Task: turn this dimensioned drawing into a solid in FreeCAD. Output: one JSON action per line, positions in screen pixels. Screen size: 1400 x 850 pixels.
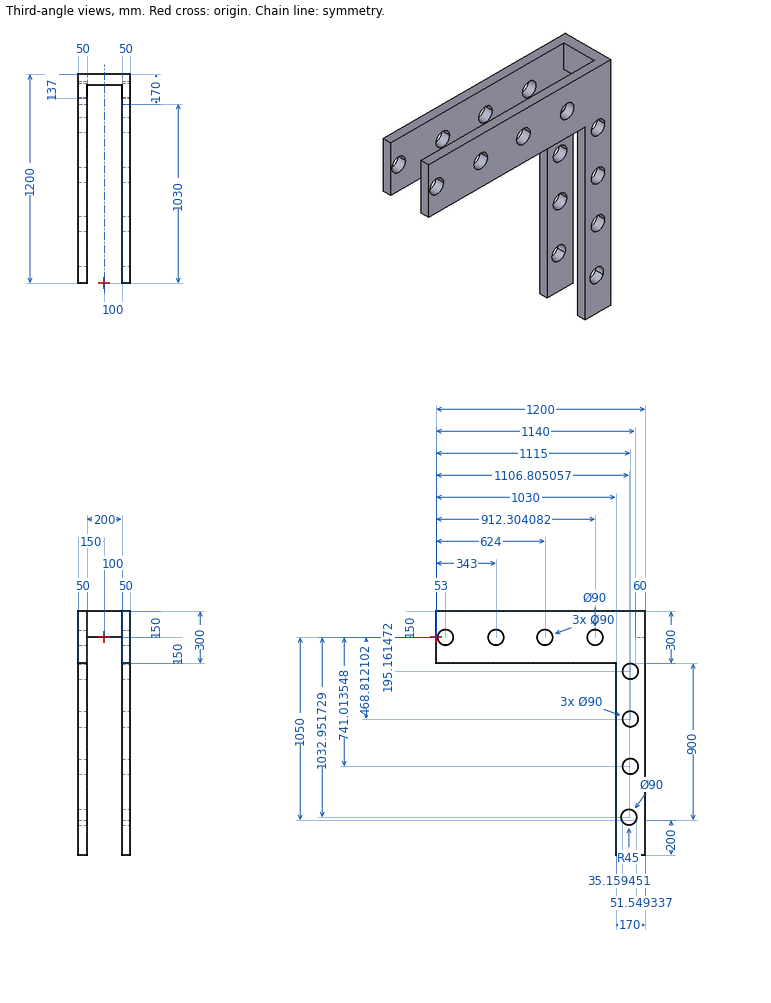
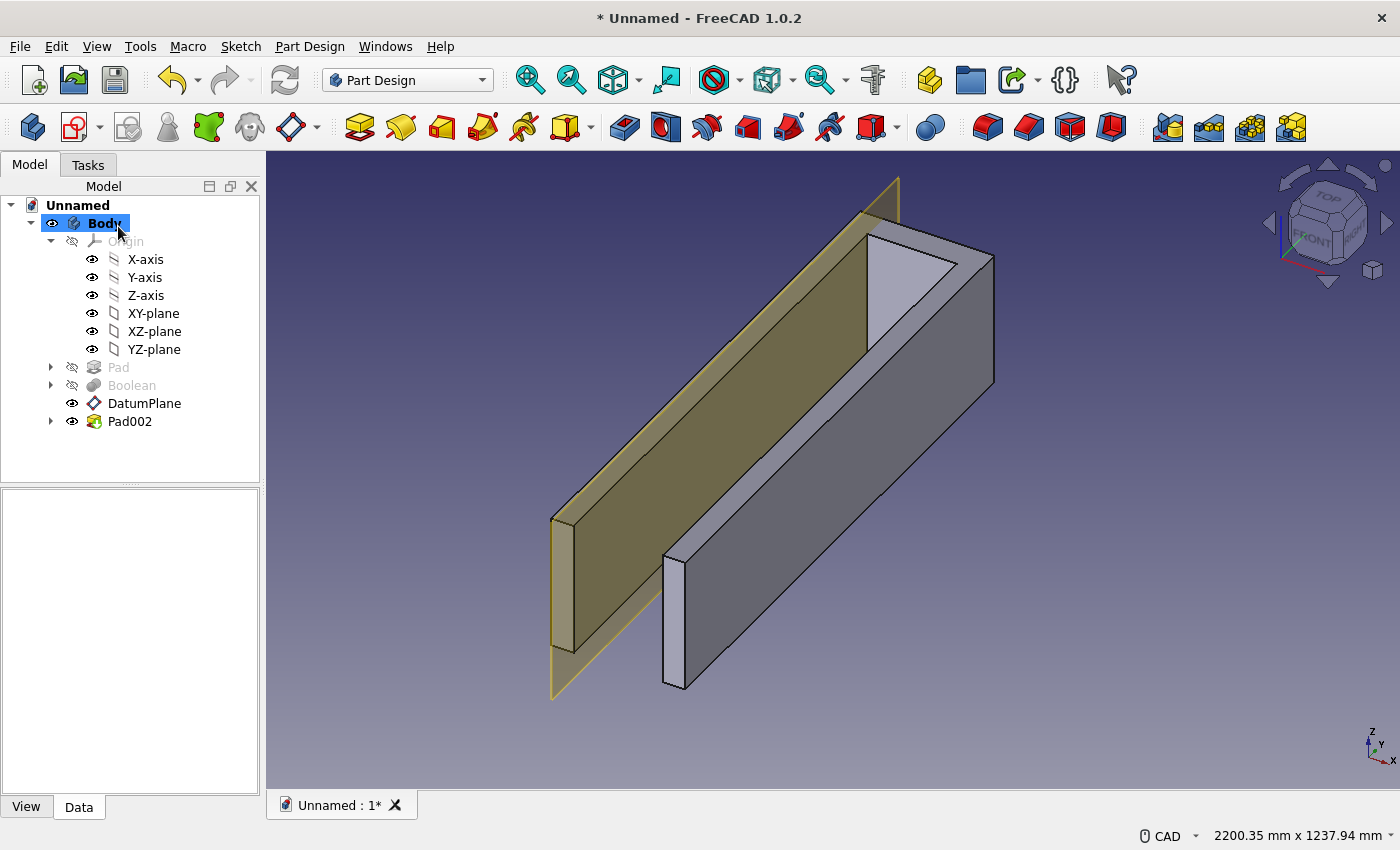
{"action": "left_click", "coordinate": [117, 403]}
{"action": "key", "text": "space"}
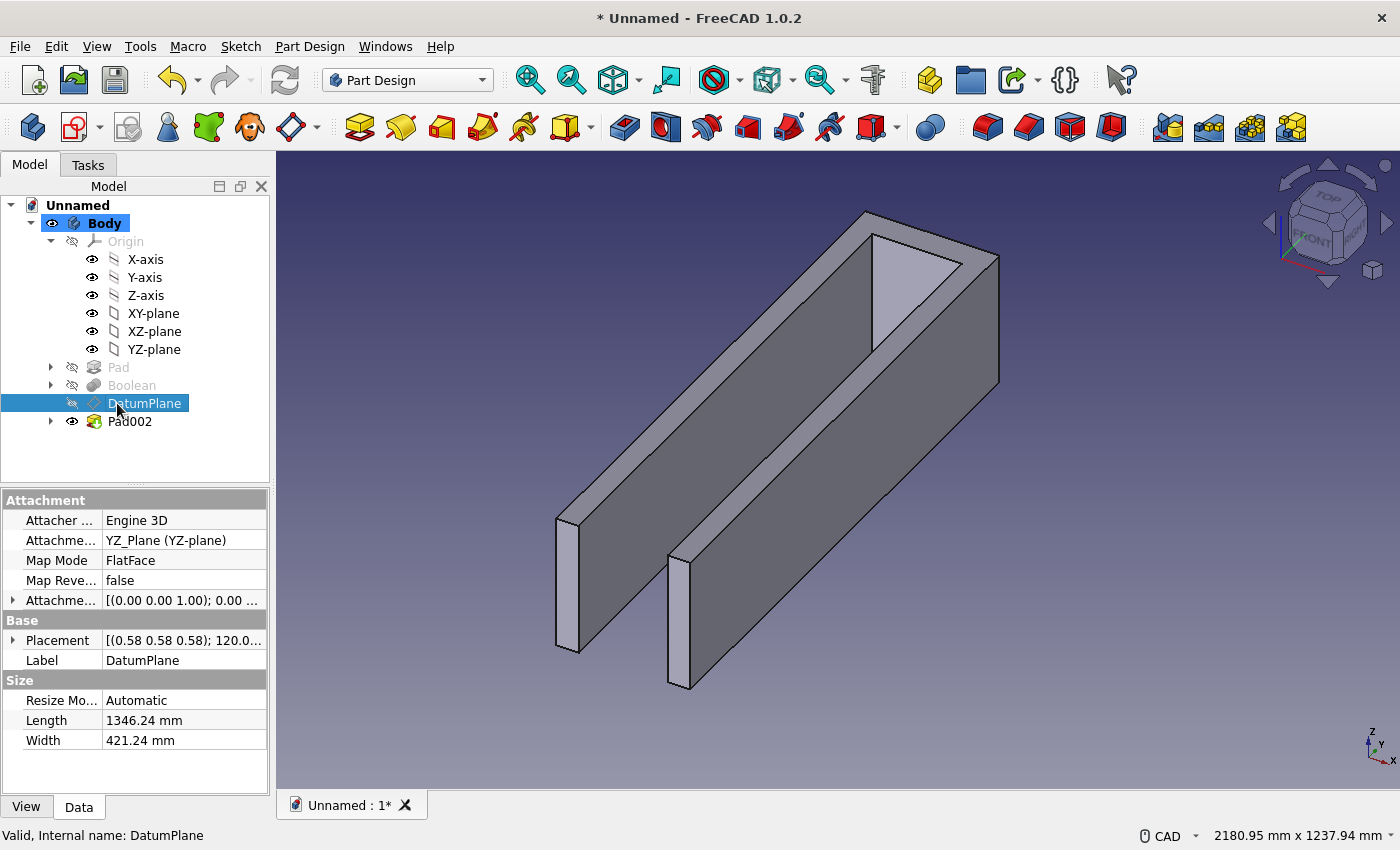
{"action": "left_click", "coordinate": [889, 428]}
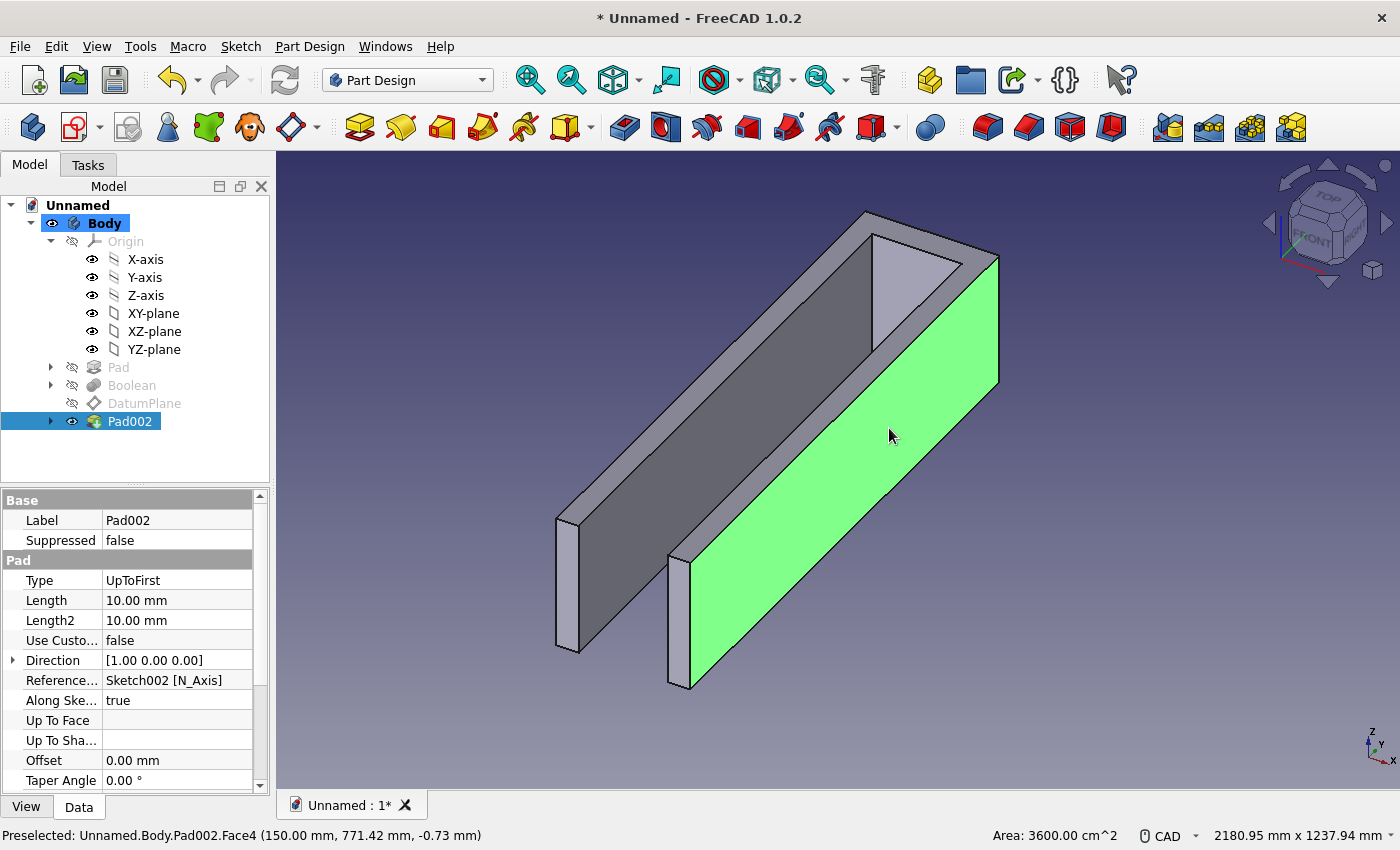
{"action": "left_click", "coordinate": [74, 128]}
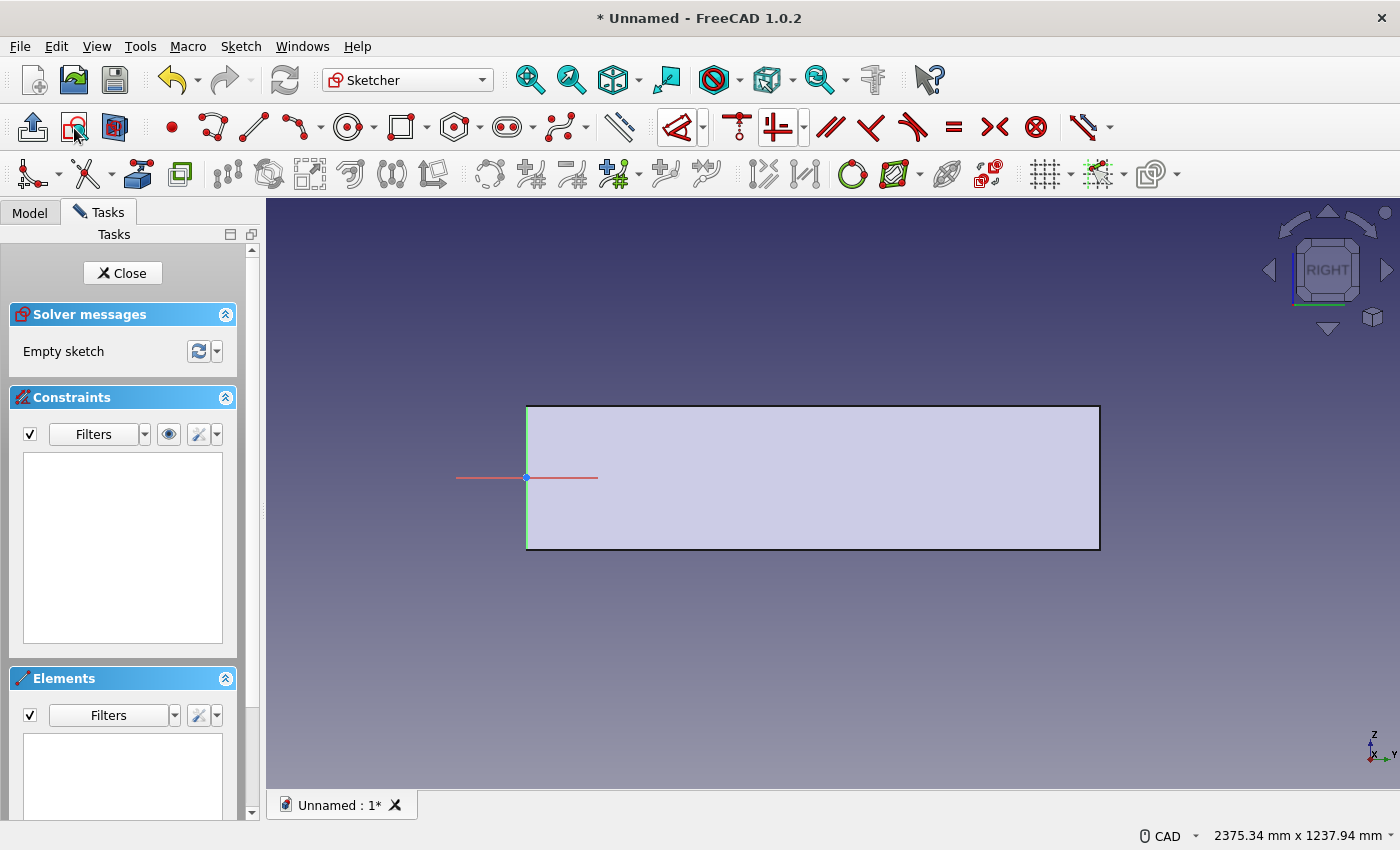
{"action": "scroll", "coordinate": [623, 465], "scroll_direction": "up", "scroll_amount": 4}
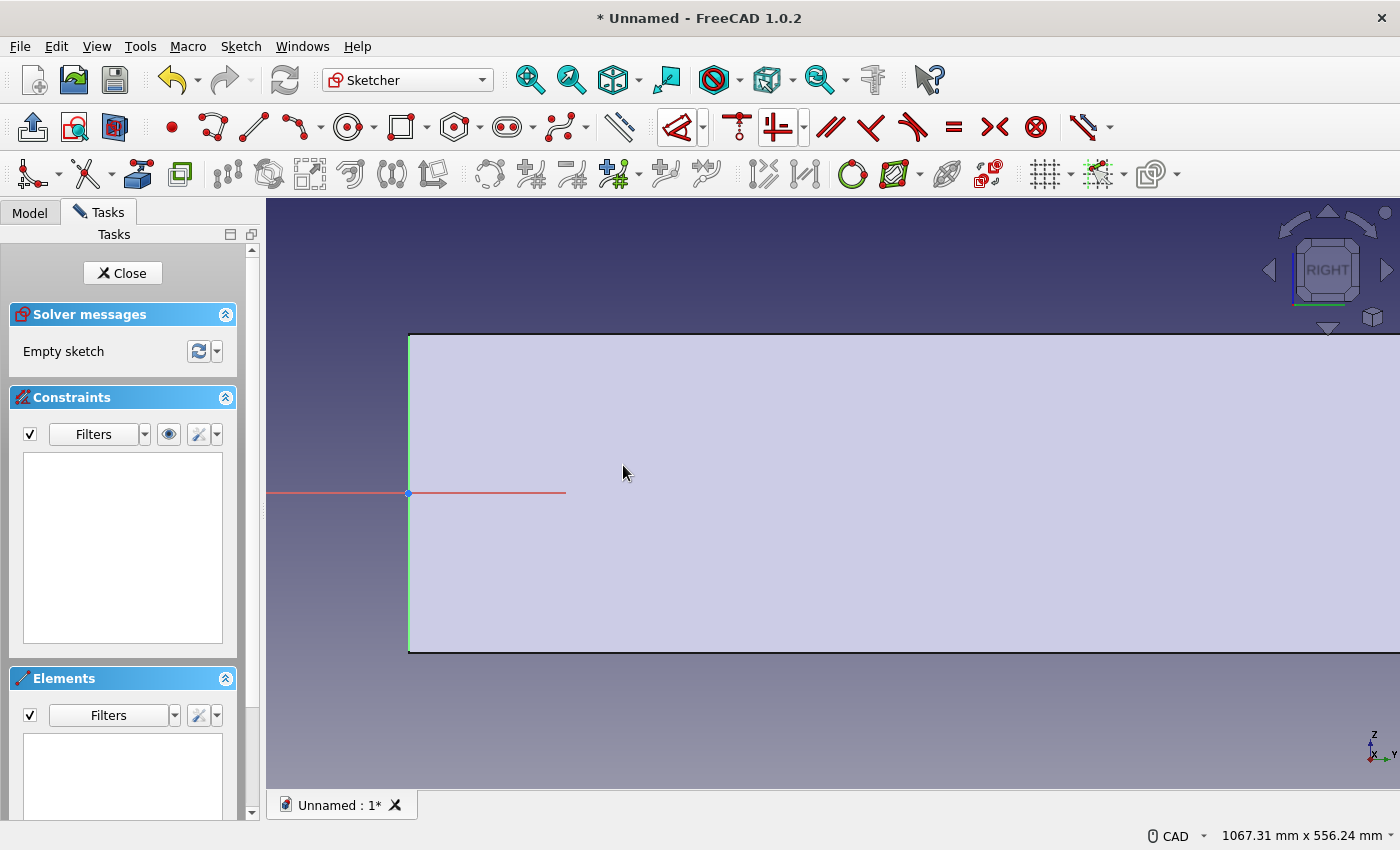
{"action": "left_click", "coordinate": [348, 128]}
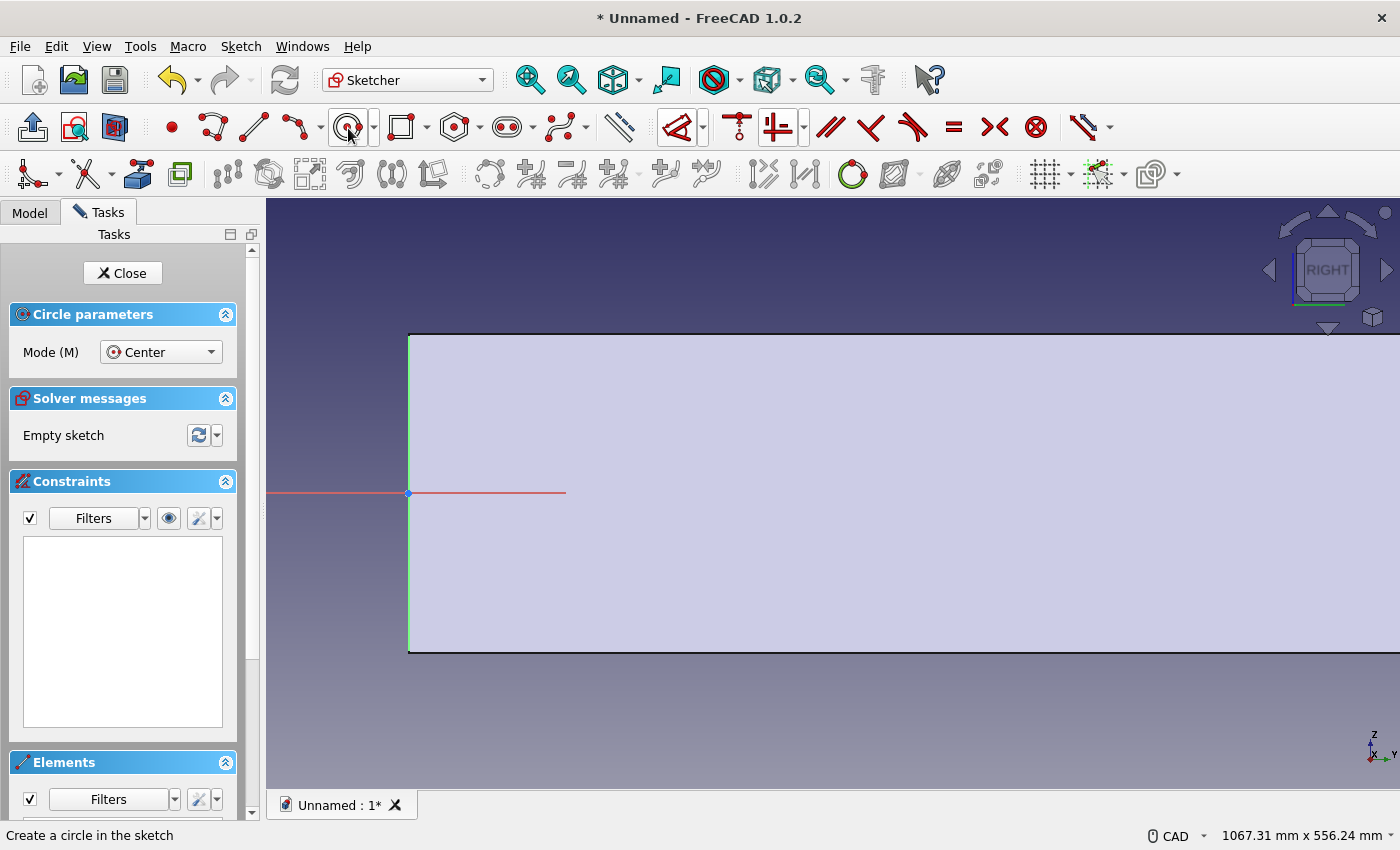
{"action": "left_click", "coordinate": [1072, 493]}
{"action": "left_click", "coordinate": [1106, 460]}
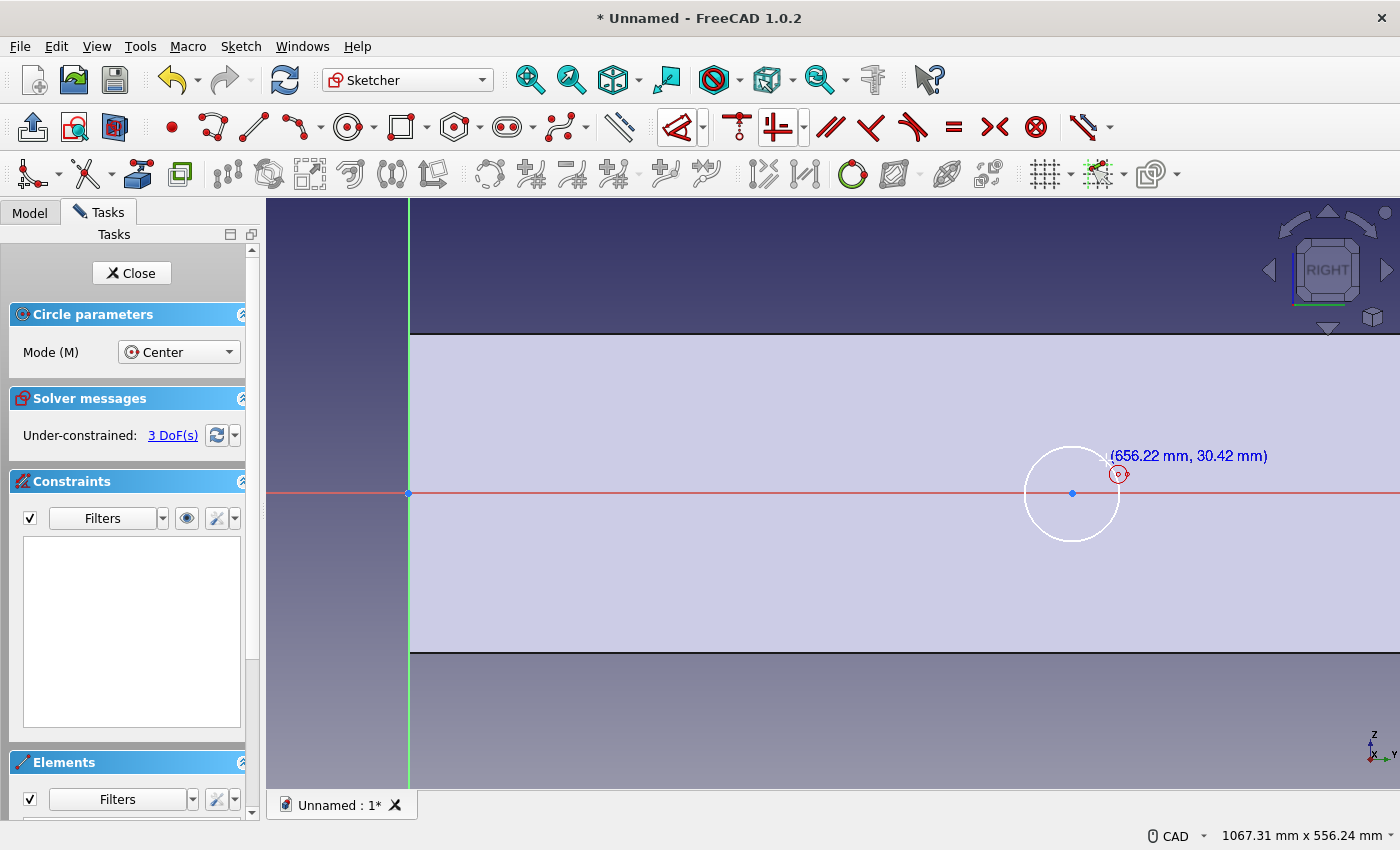
{"action": "left_click", "coordinate": [773, 493]}
{"action": "left_click", "coordinate": [807, 460]}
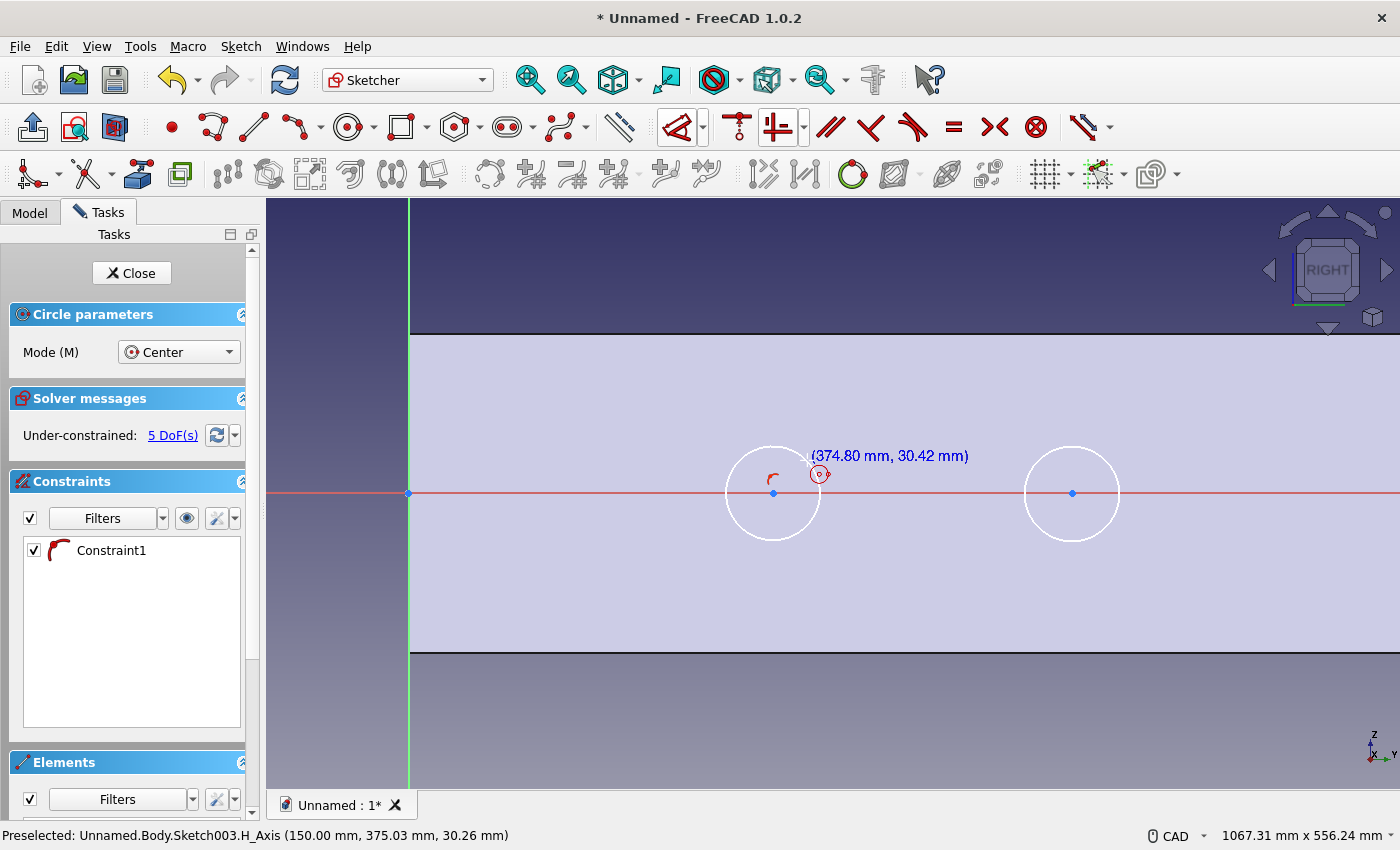
{"action": "left_click", "coordinate": [465, 493]}
{"action": "left_click", "coordinate": [499, 460]}
{"action": "key", "text": "Escape"}